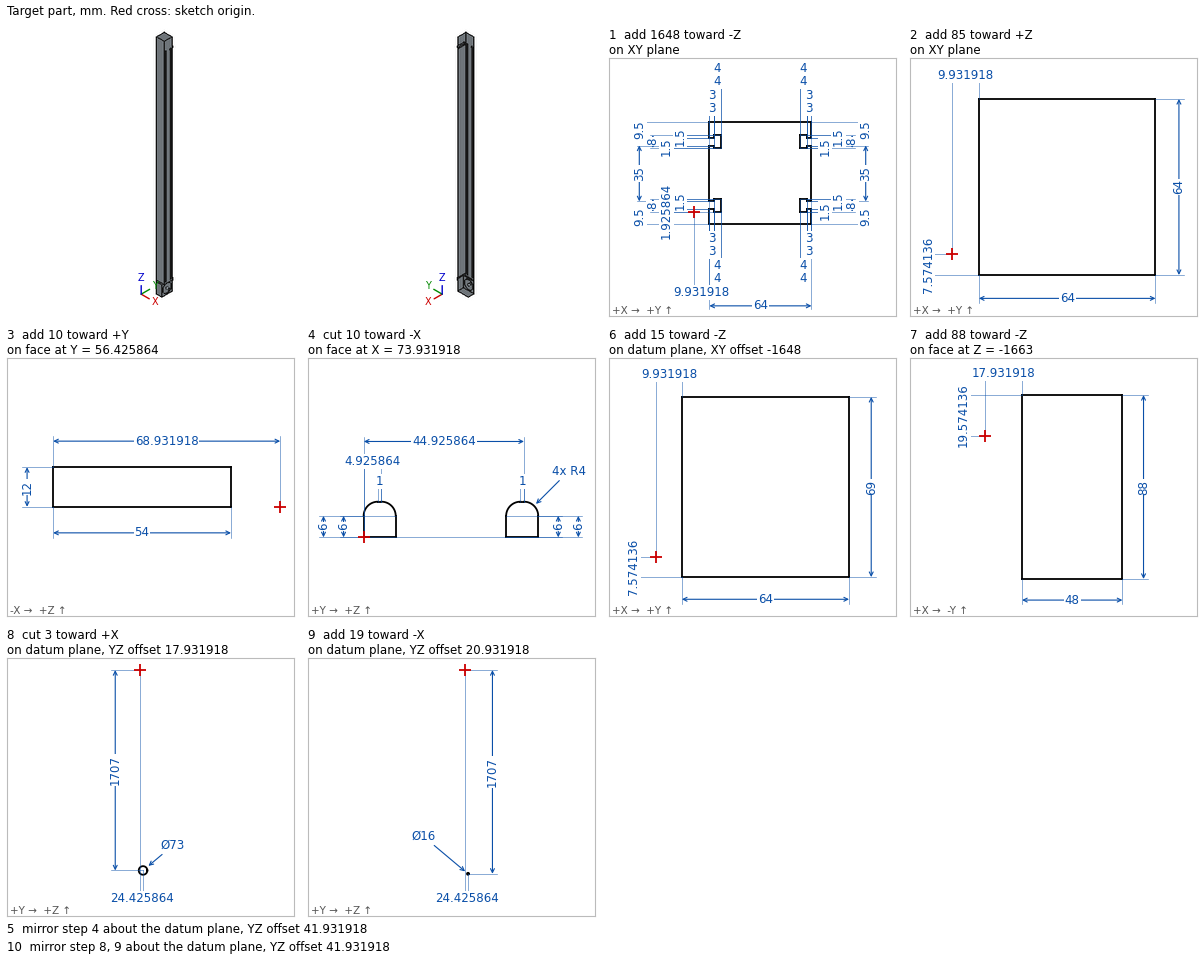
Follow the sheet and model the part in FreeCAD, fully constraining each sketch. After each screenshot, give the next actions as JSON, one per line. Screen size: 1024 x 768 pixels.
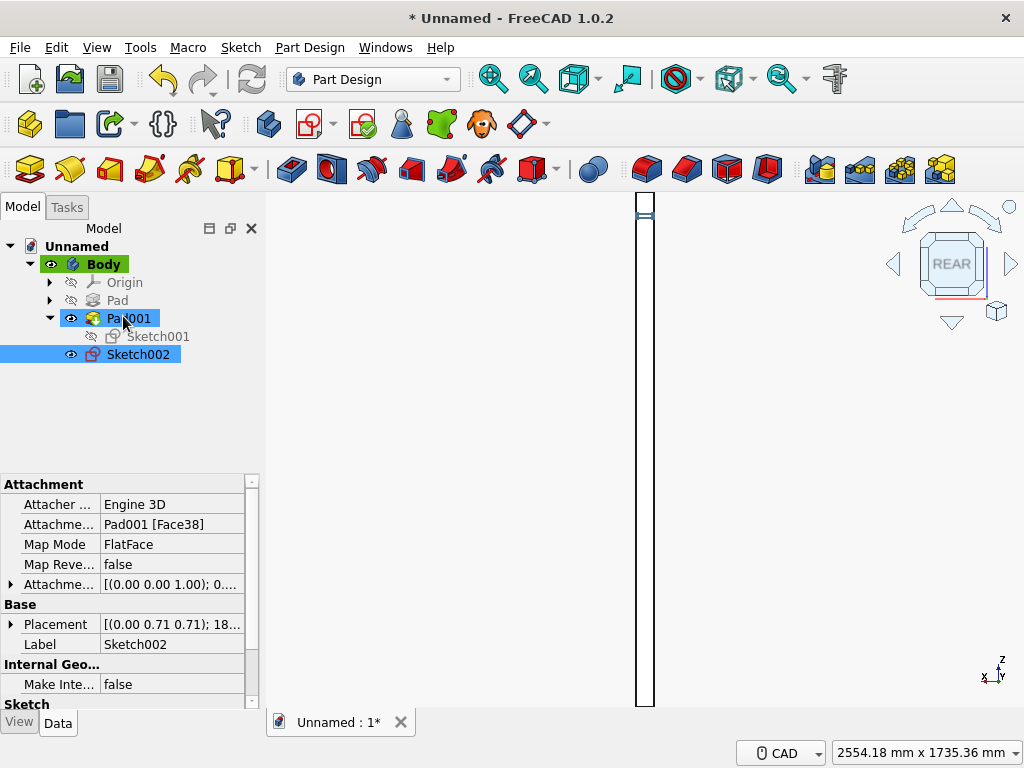
{"action": "left_click", "coordinate": [30, 170]}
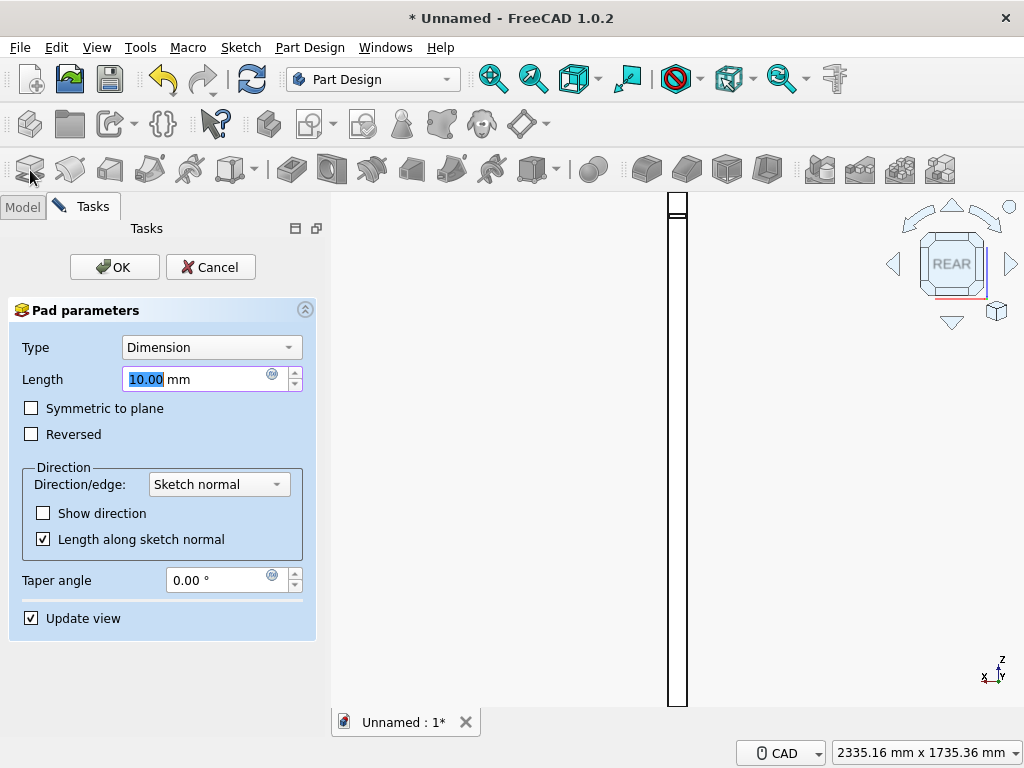
{"action": "type", "text": "10"}
{"action": "key", "text": "Tab"}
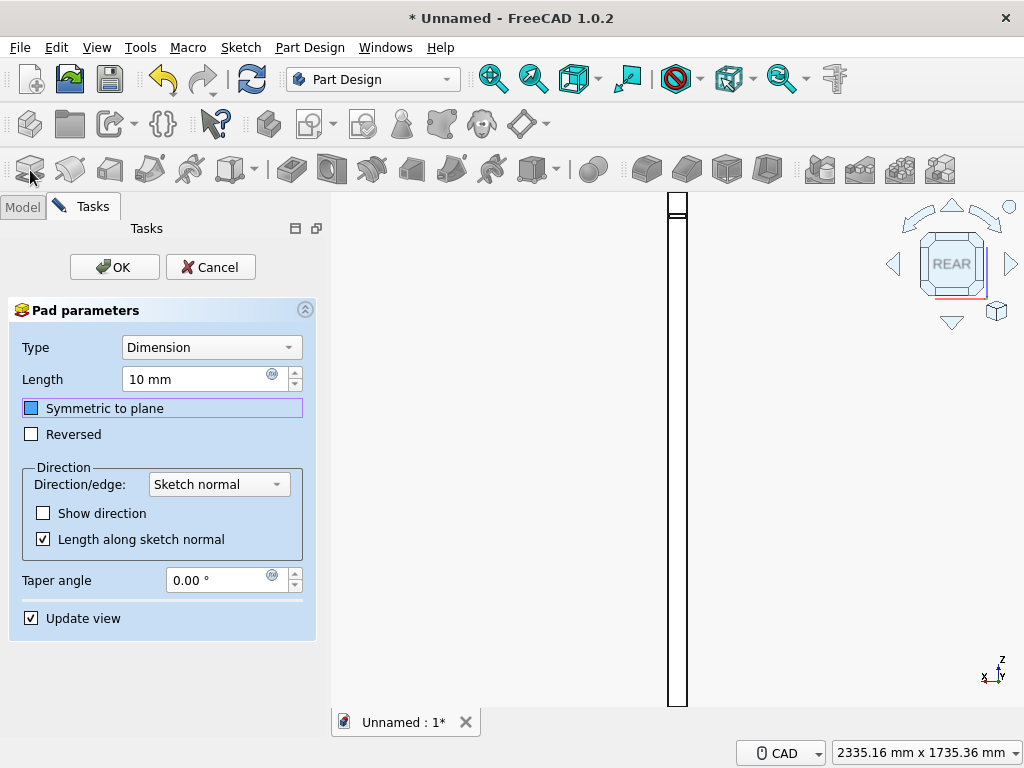
{"action": "left_click", "coordinate": [115, 267]}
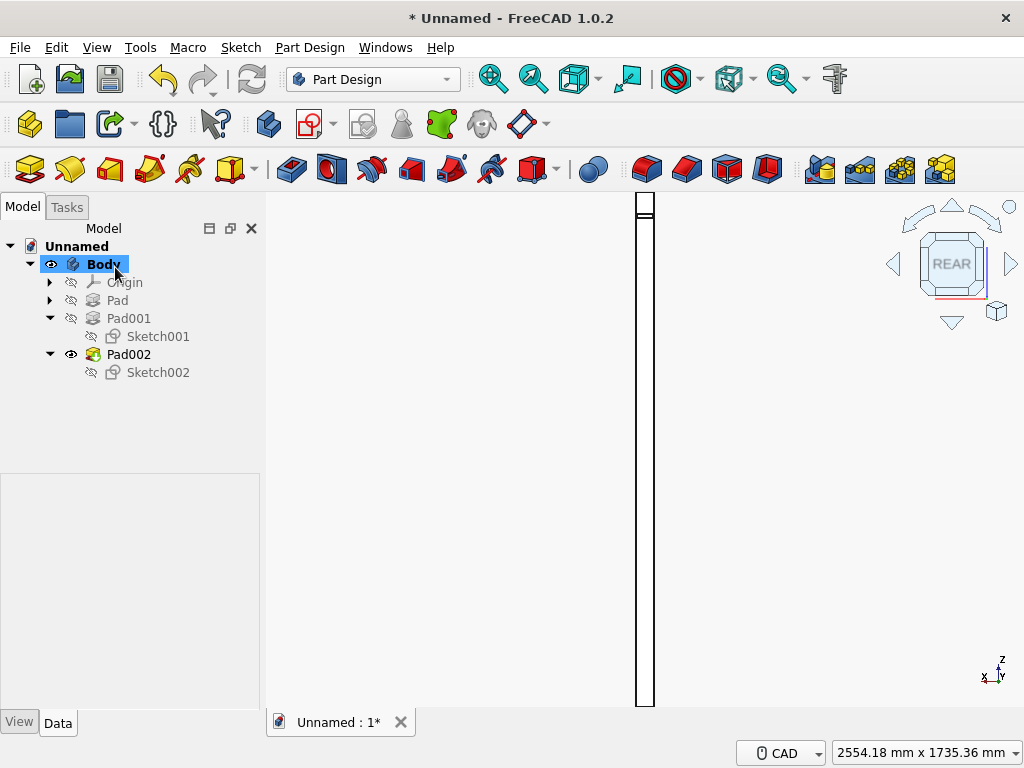
{"action": "left_click", "coordinate": [494, 80]}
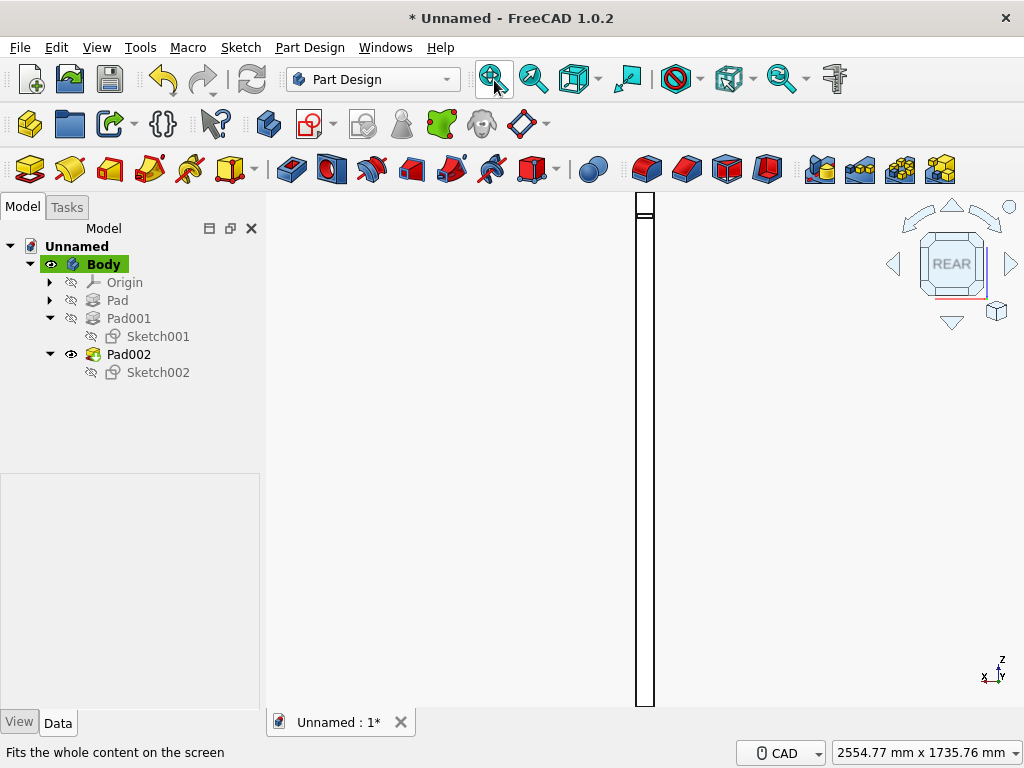
{"action": "key", "text": "0"}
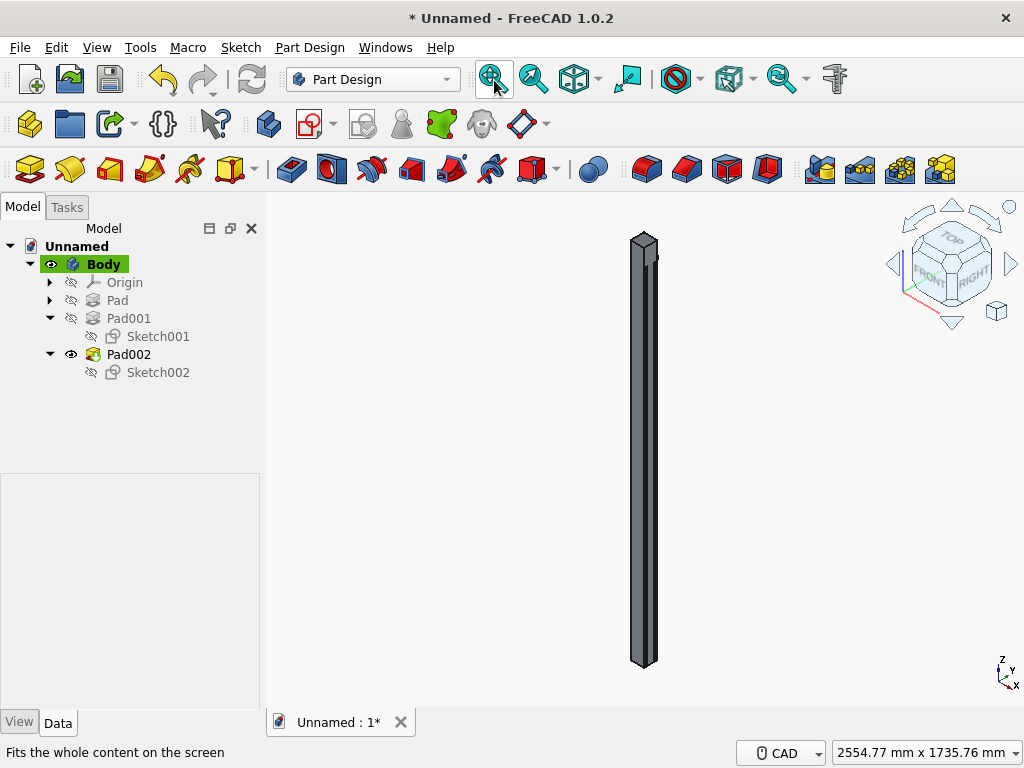
{"action": "scroll", "coordinate": [651, 273], "scroll_direction": "up", "scroll_amount": 5}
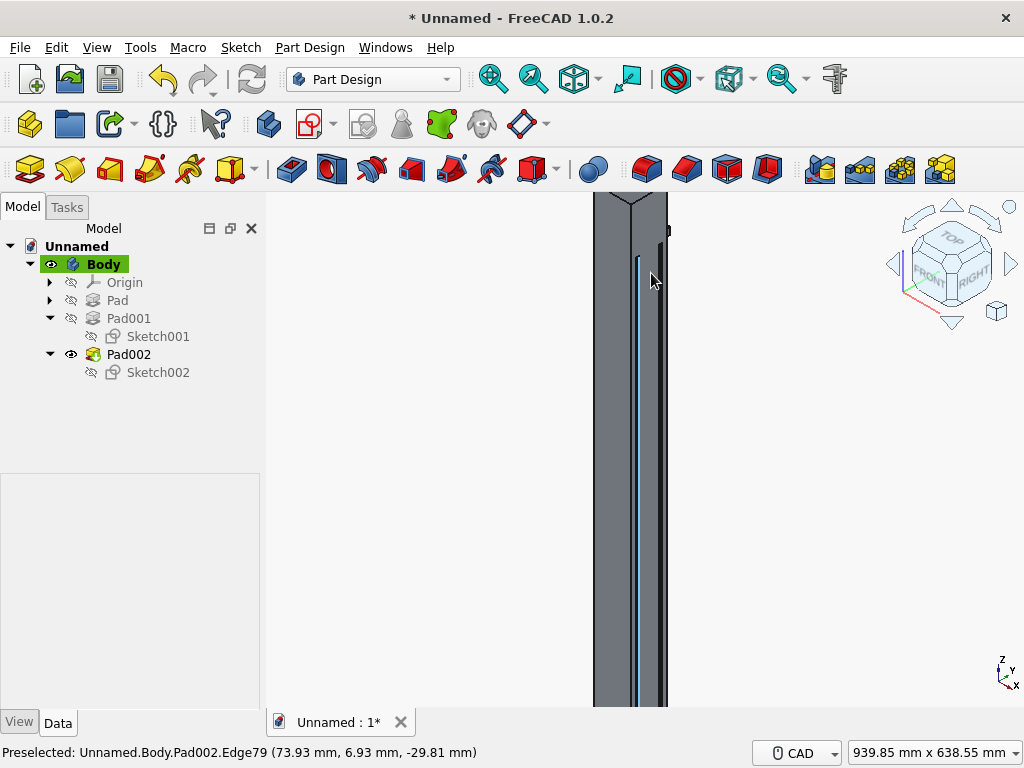
{"action": "left_click", "coordinate": [649, 275]}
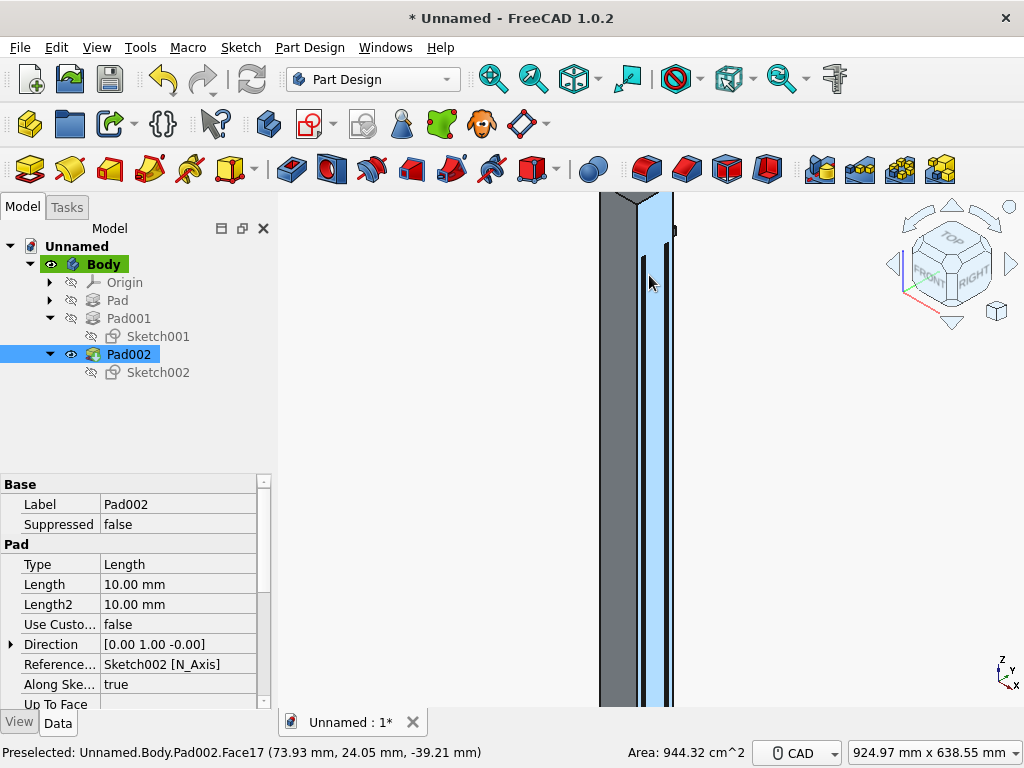
{"action": "left_click", "coordinate": [310, 124]}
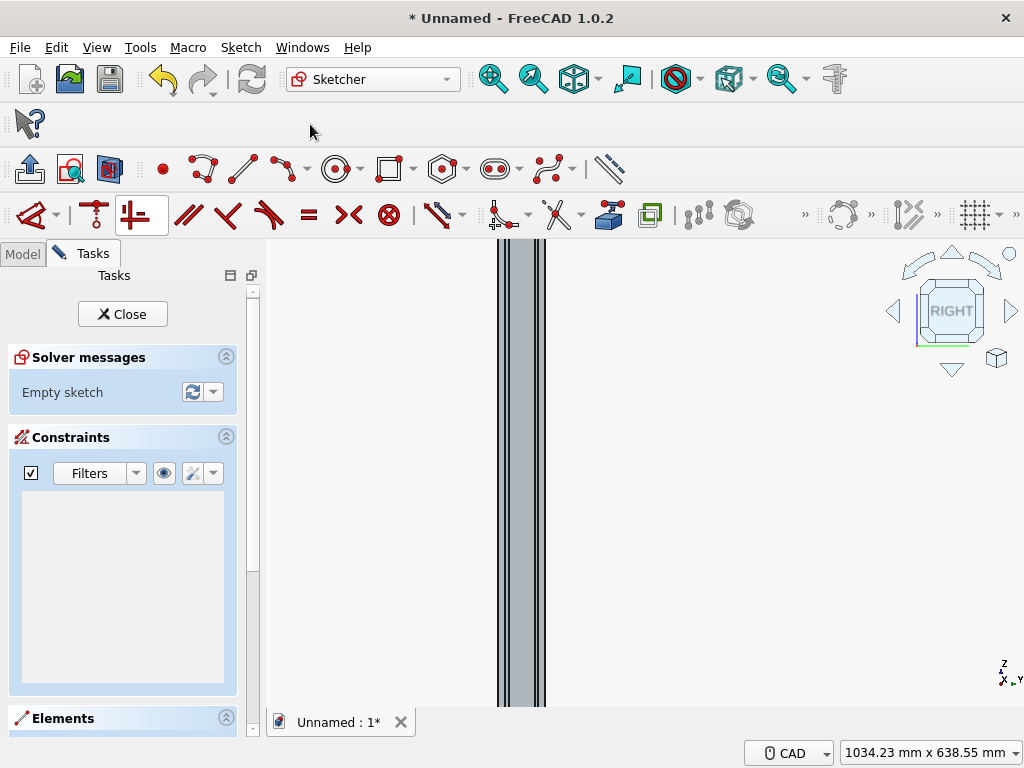
{"action": "scroll", "coordinate": [576, 473], "scroll_direction": "down", "scroll_amount": 5}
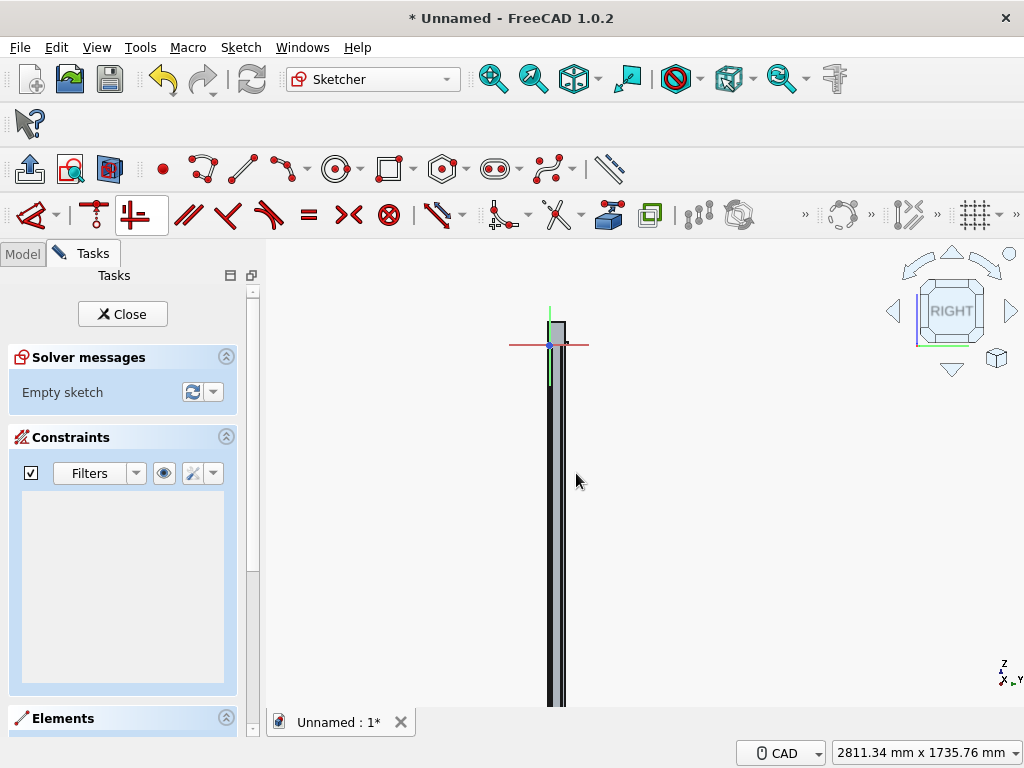
{"action": "scroll", "coordinate": [555, 337], "scroll_direction": "up", "scroll_amount": 15}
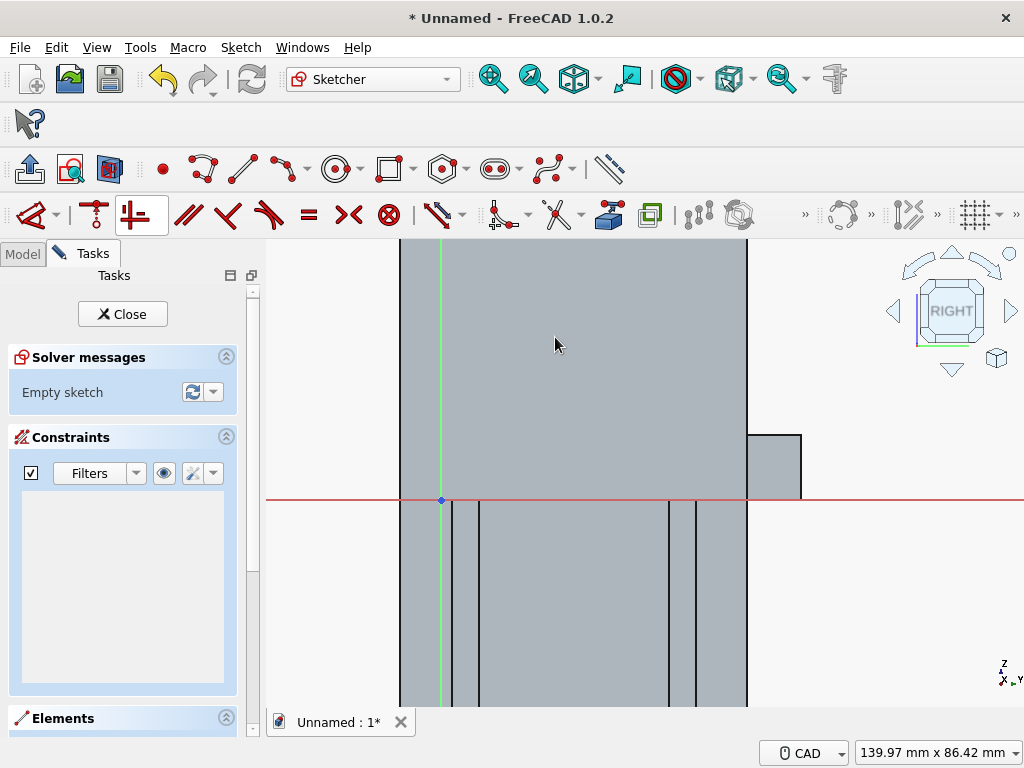
{"action": "scroll", "coordinate": [568, 473], "scroll_direction": "up", "scroll_amount": 2}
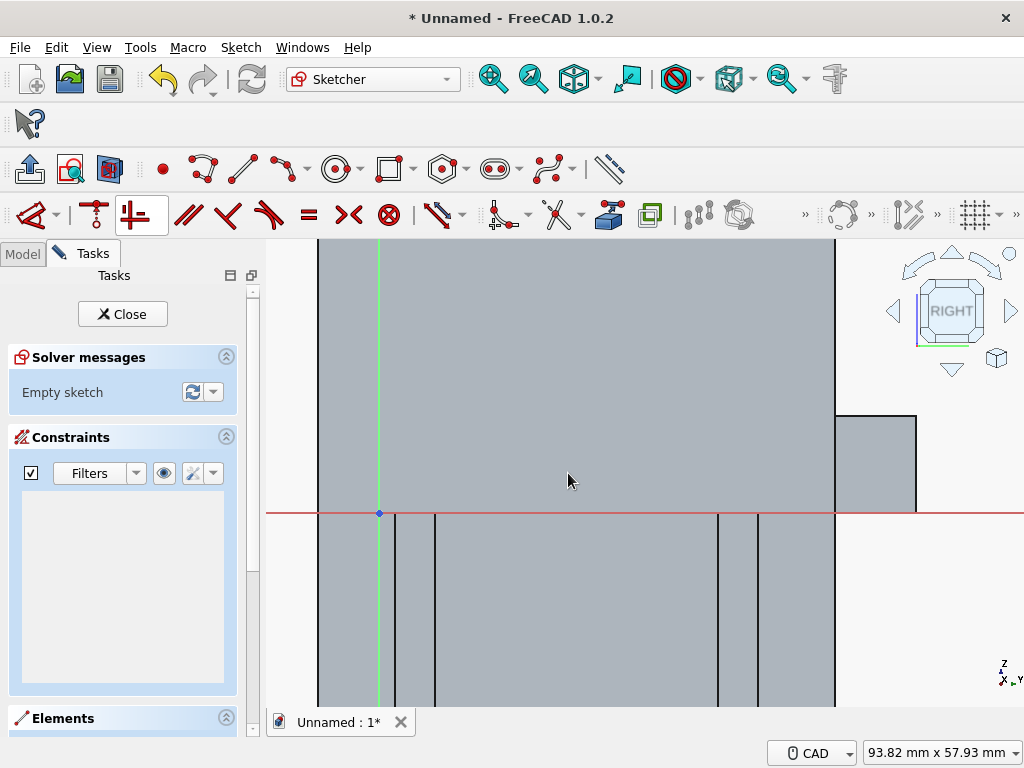
{"action": "left_click", "coordinate": [244, 170]}